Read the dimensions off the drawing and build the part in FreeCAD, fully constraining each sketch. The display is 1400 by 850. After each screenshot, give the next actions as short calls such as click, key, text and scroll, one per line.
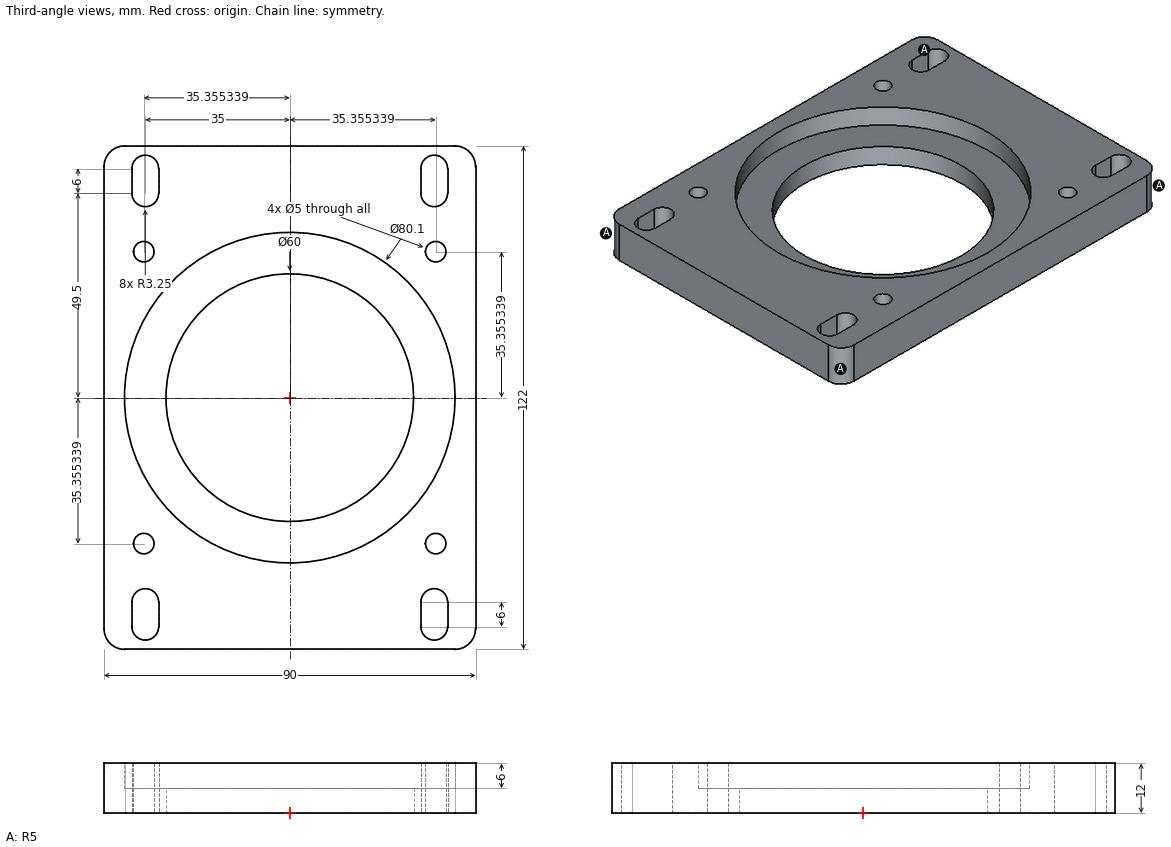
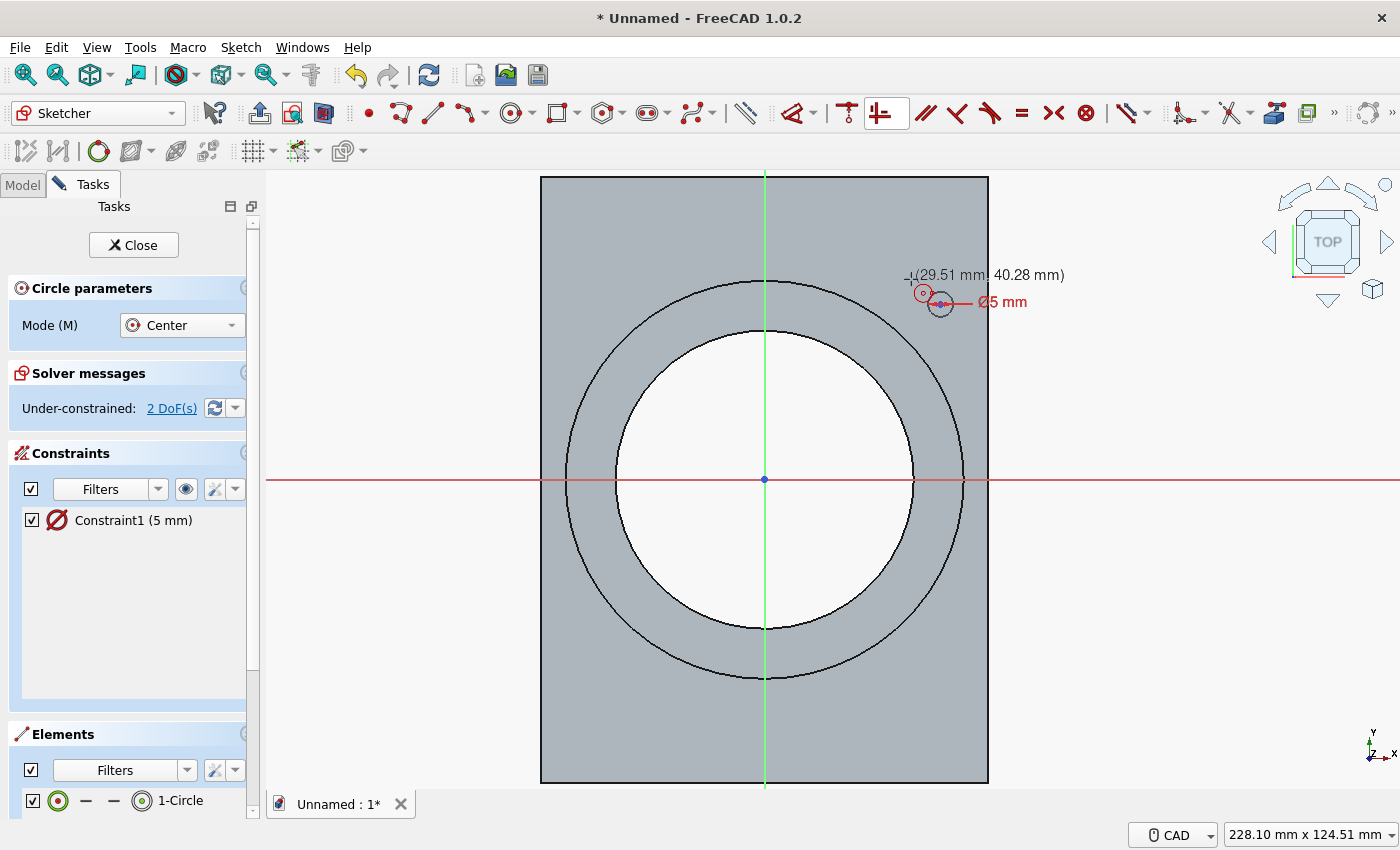
scroll(589, 304, up, 4)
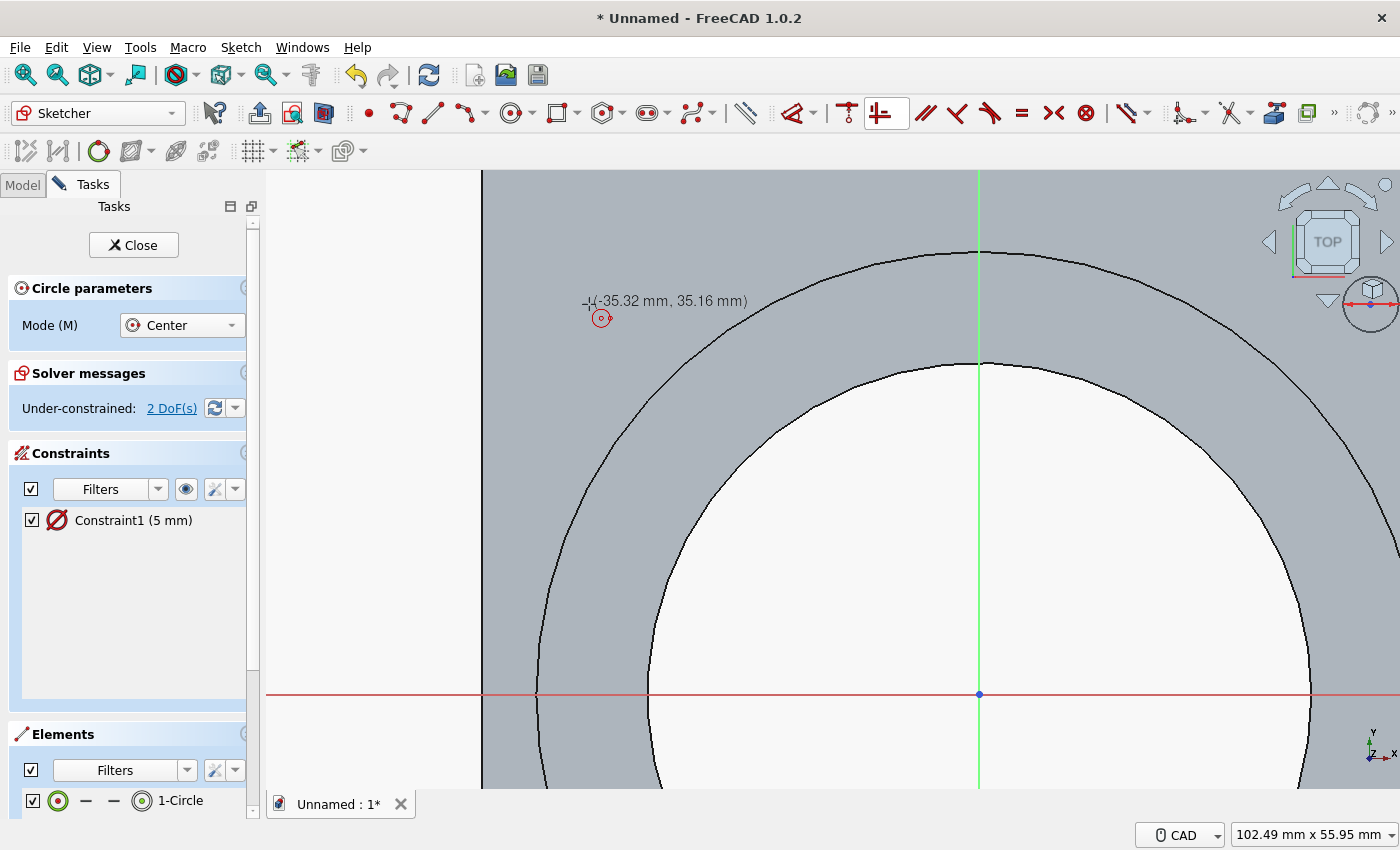
click(588, 304)
move(608, 284)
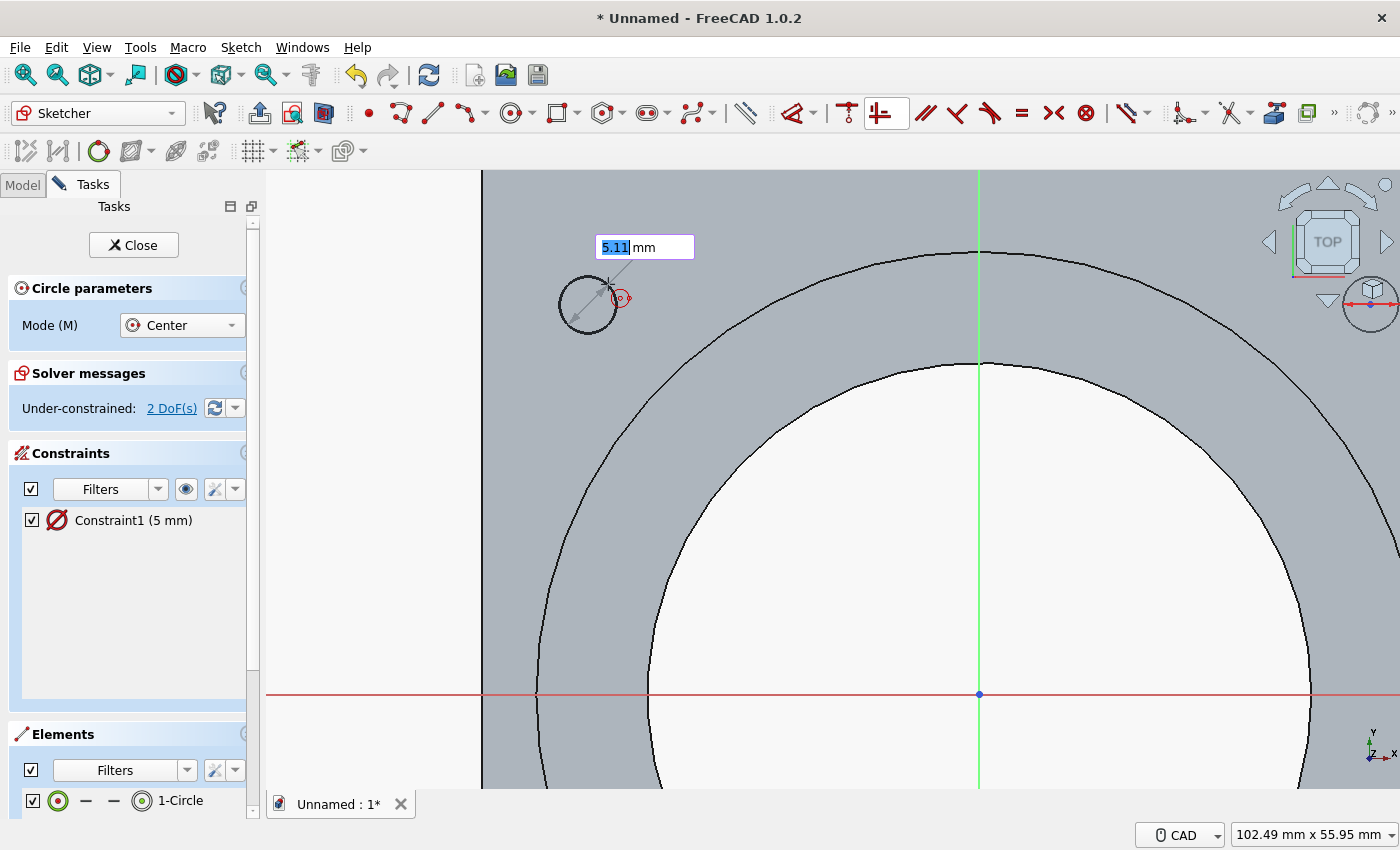
text(5)
key(Return)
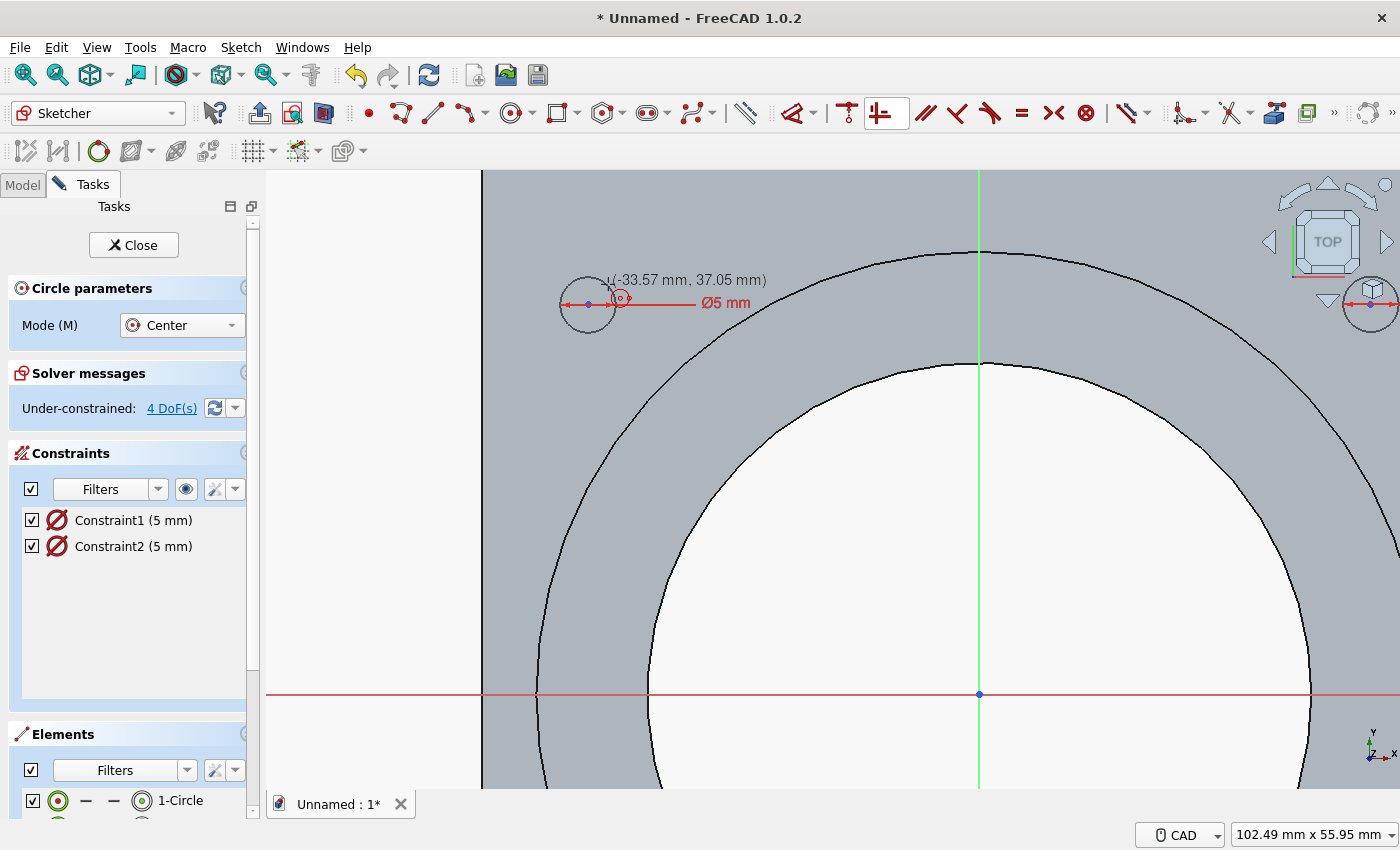
scroll(589, 304, down, 4)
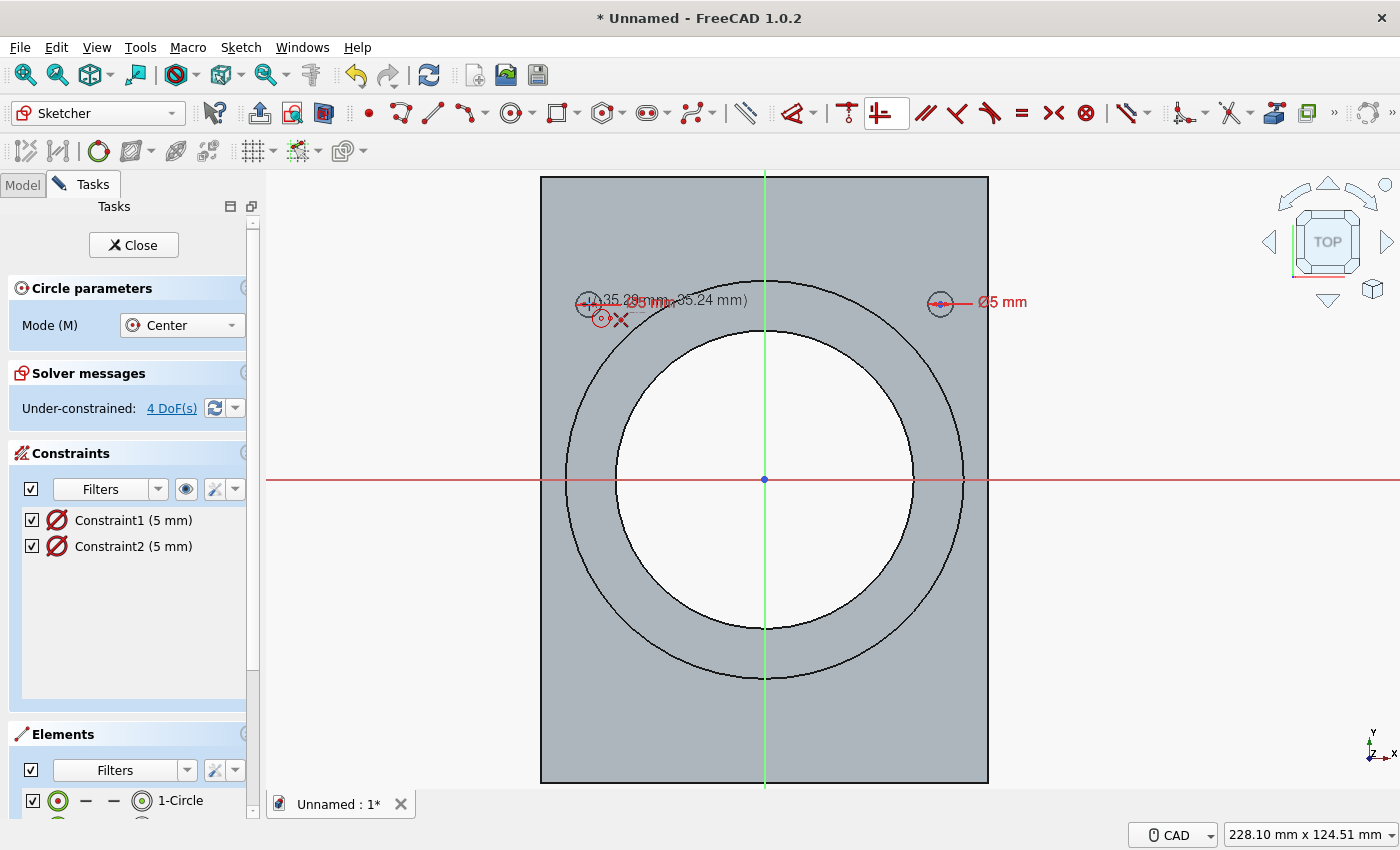
scroll(589, 656, up, 4)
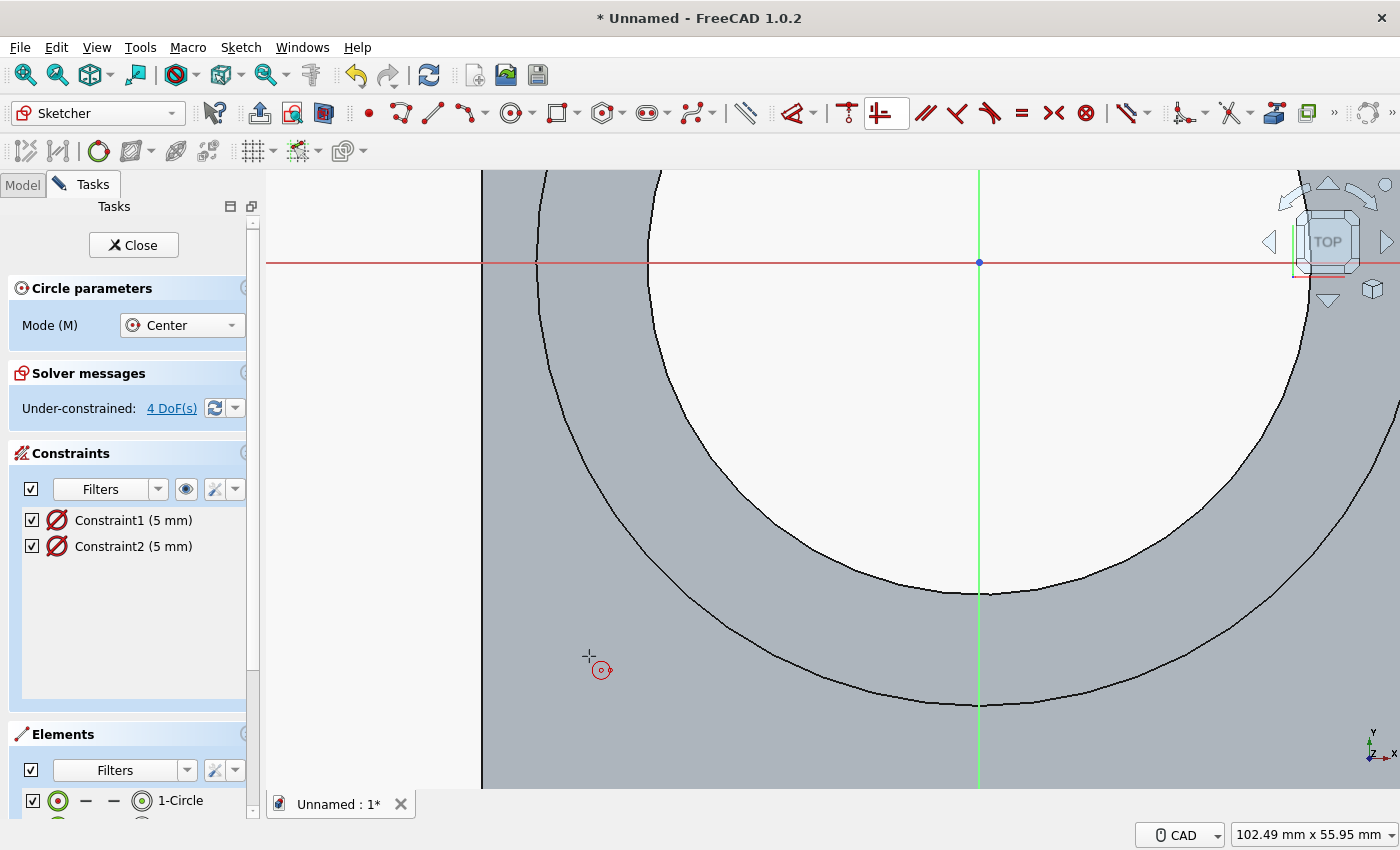
click(588, 654)
move(608, 634)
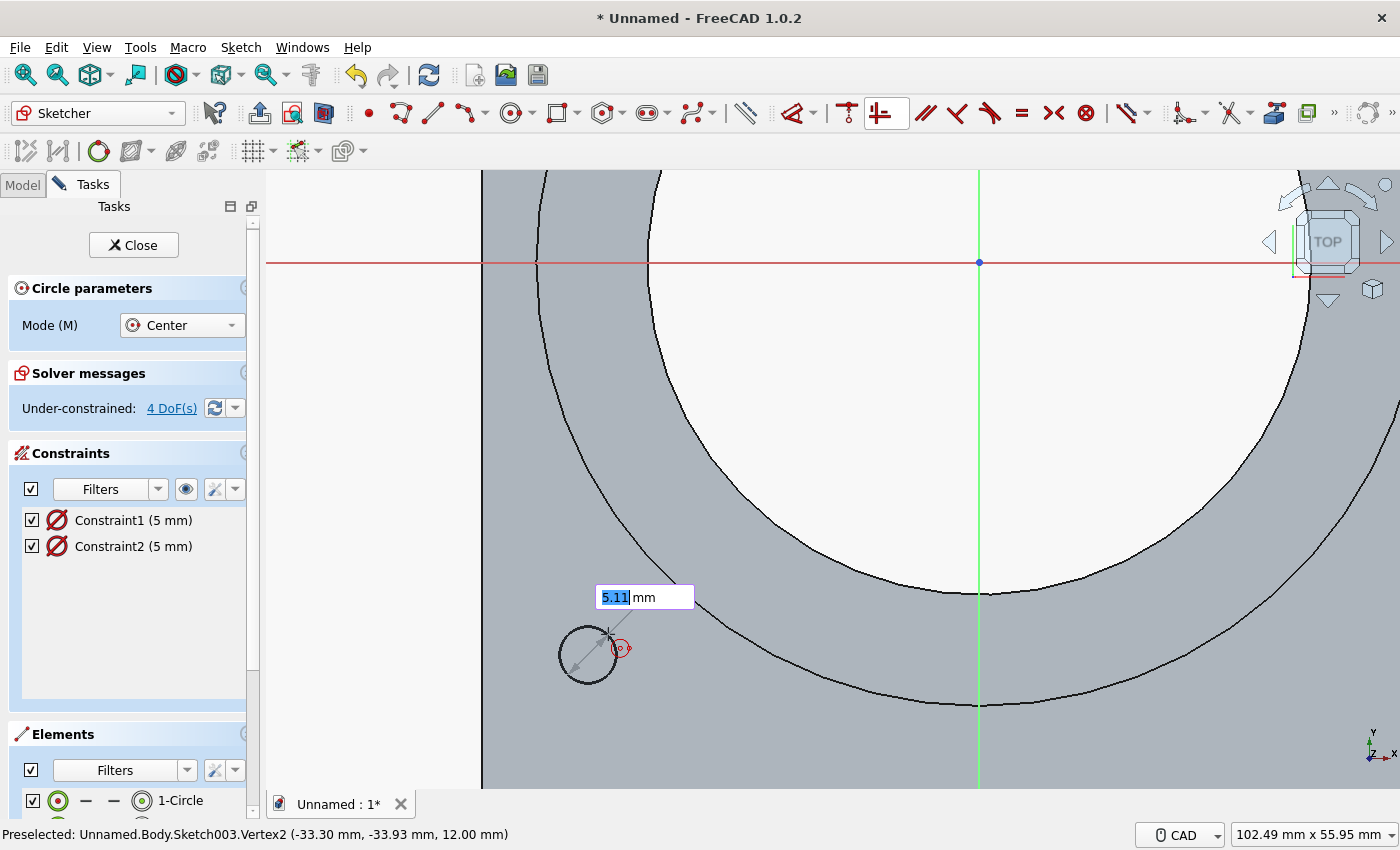
text(5)
key(Return)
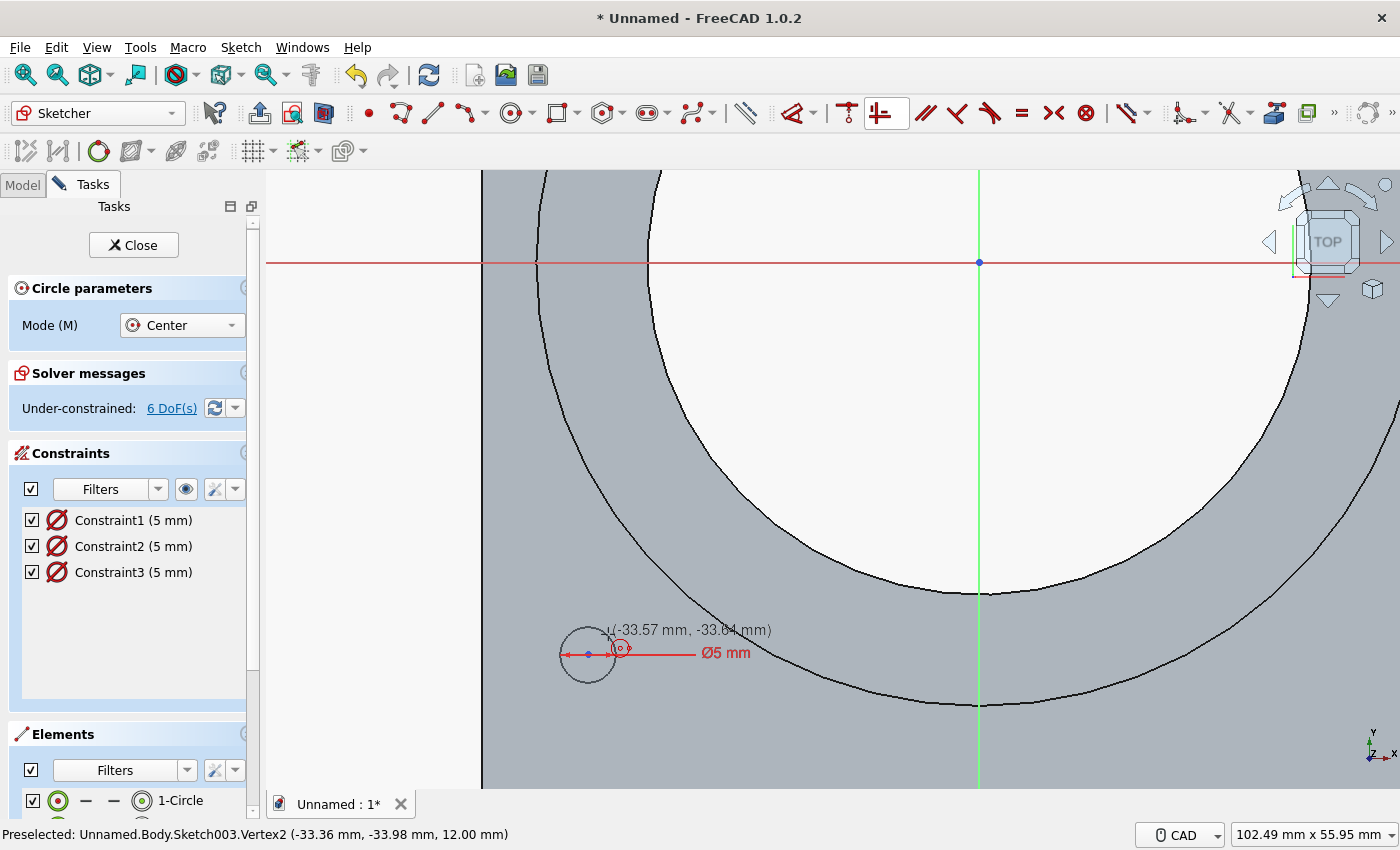
scroll(589, 656, down, 4)